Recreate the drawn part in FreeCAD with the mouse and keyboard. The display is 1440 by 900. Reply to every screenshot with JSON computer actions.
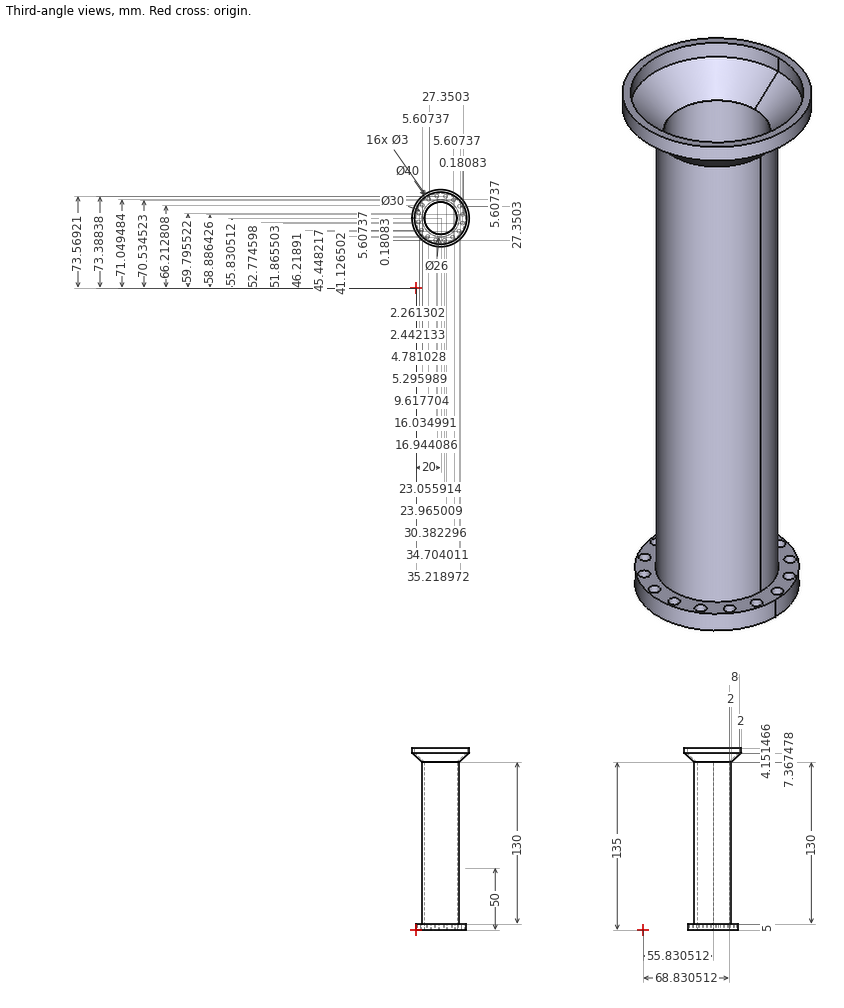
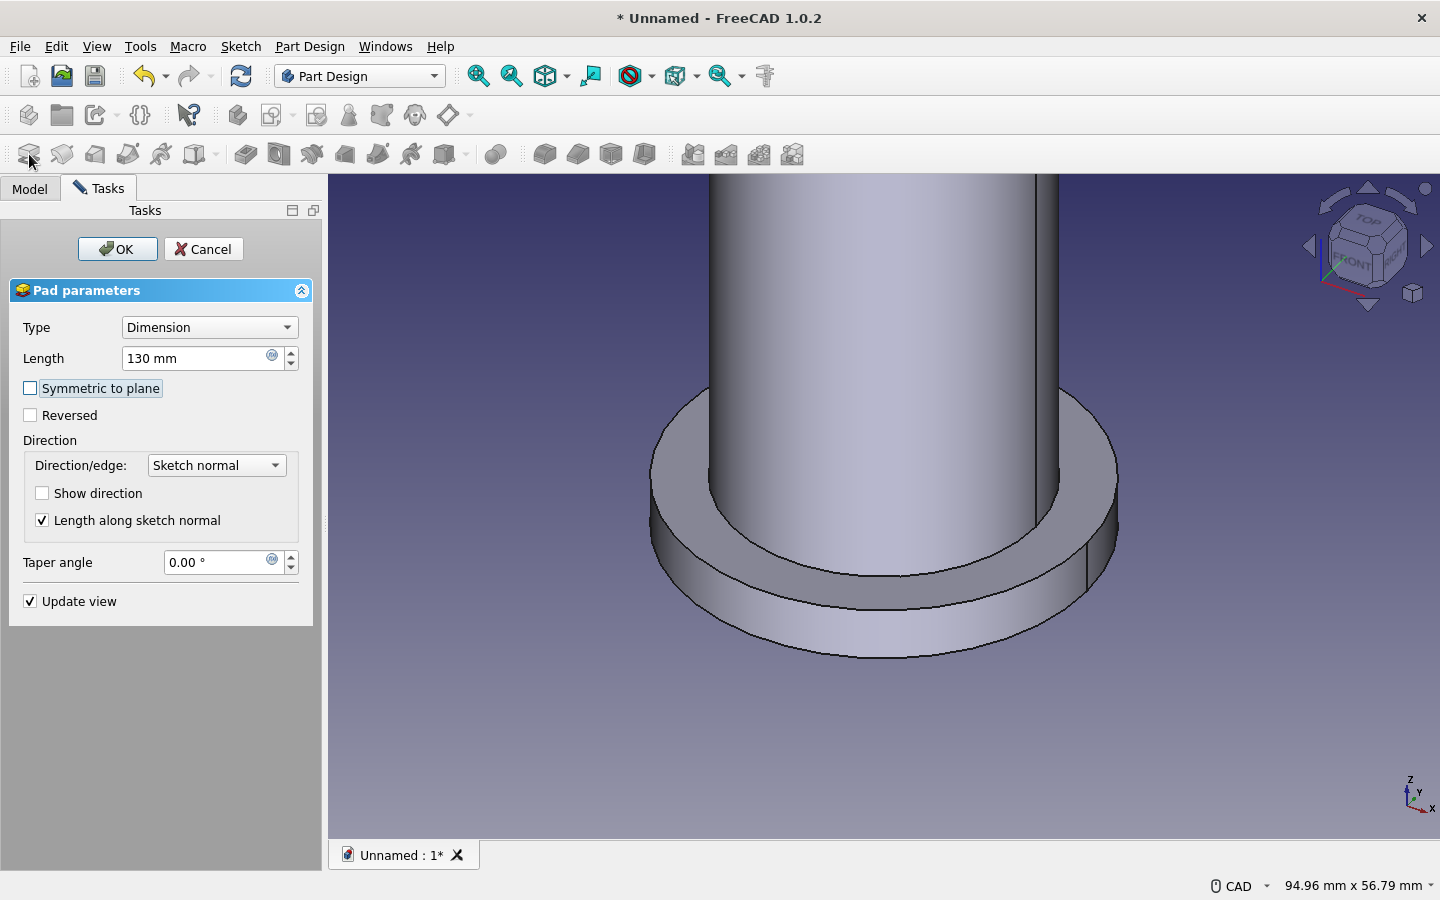
{"action": "left_click", "coordinate": [118, 249]}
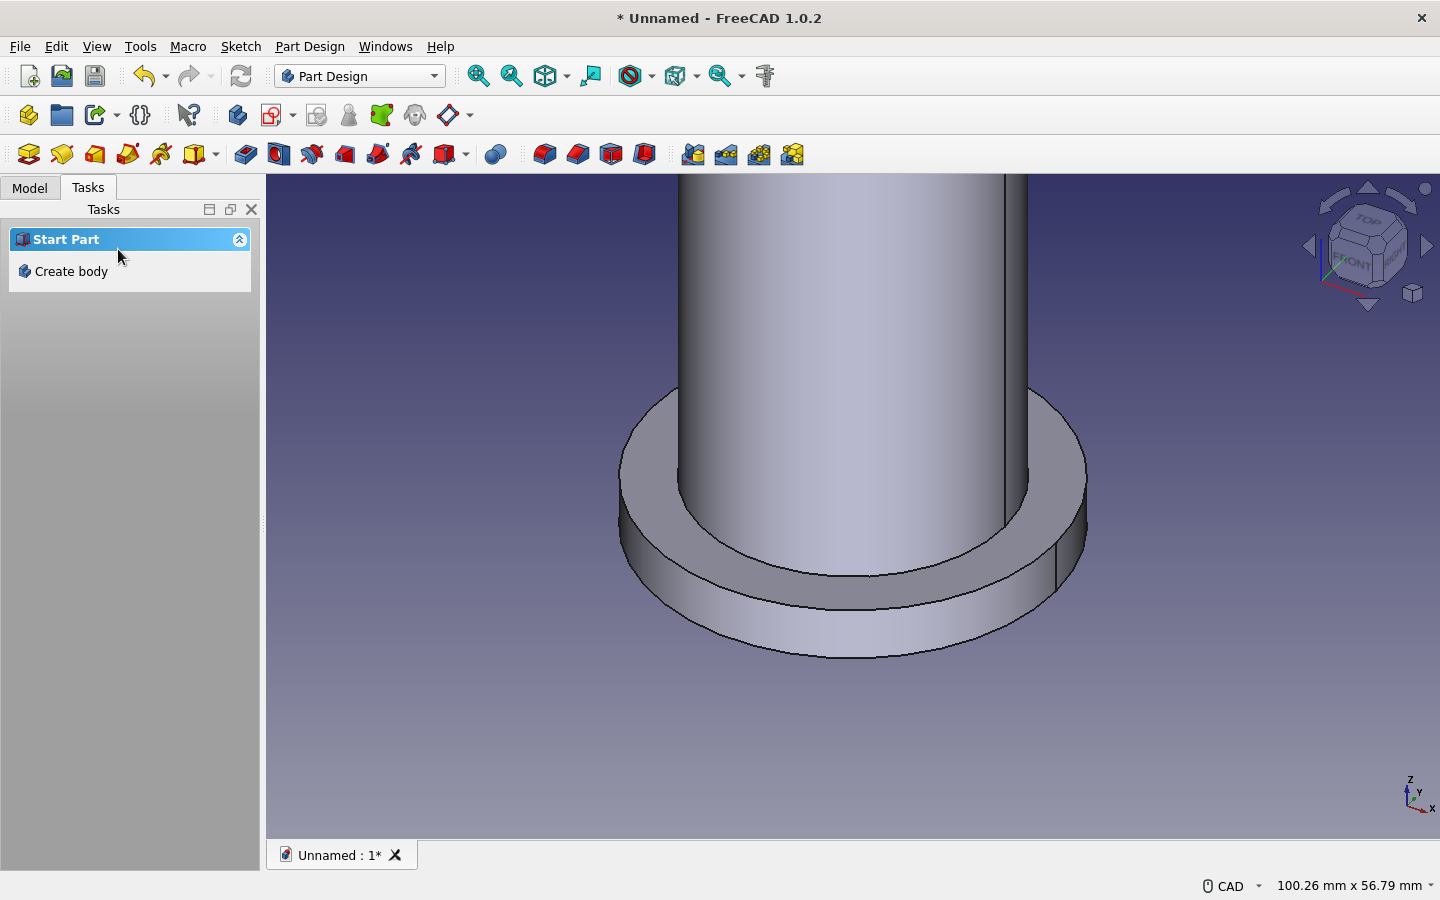
{"action": "left_click", "coordinate": [479, 76]}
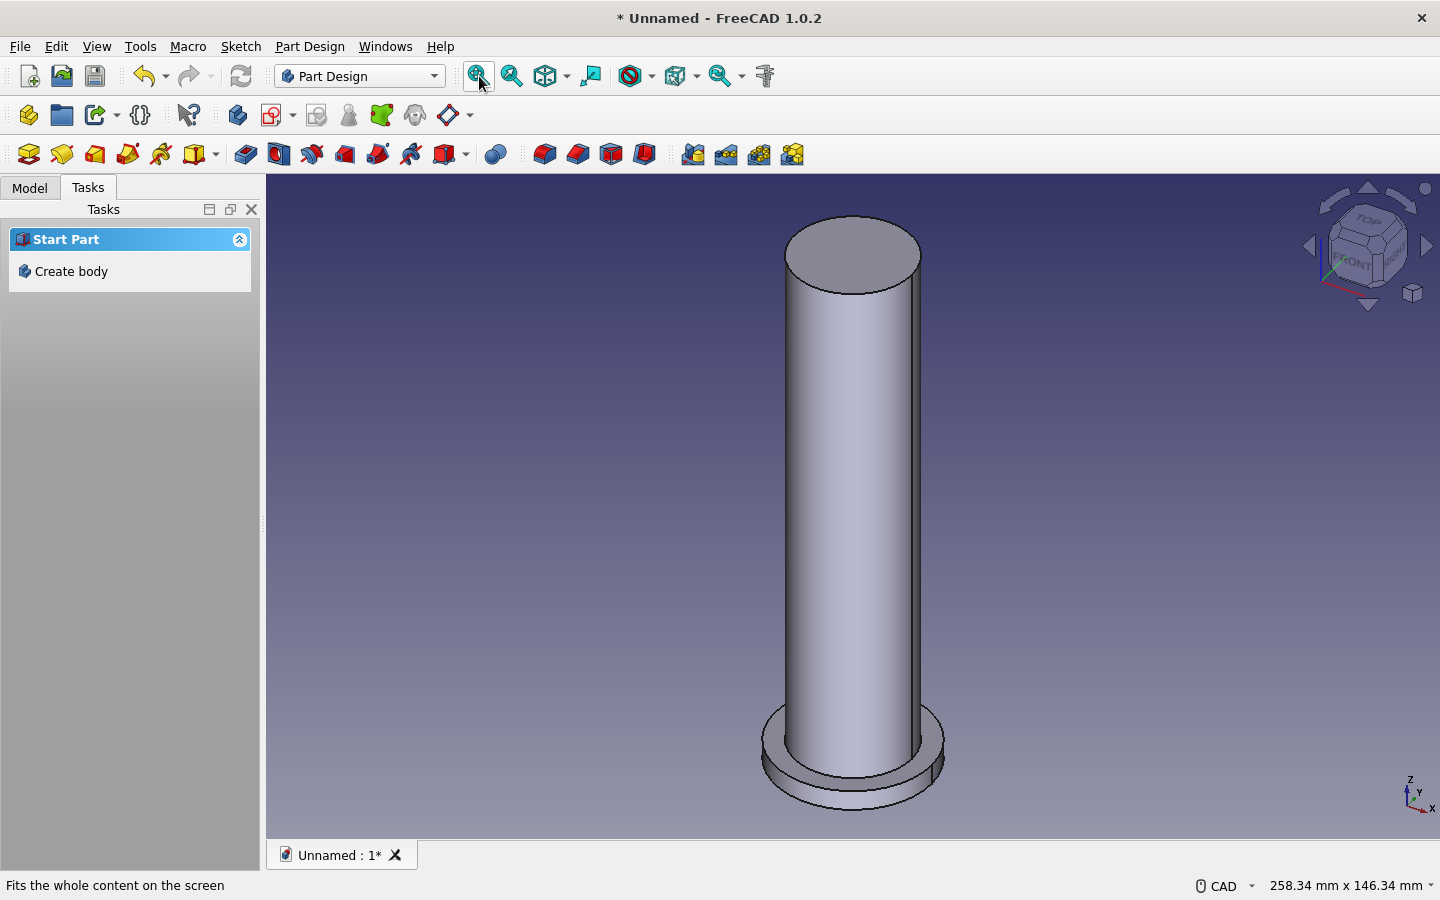
{"action": "left_click", "coordinate": [853, 254]}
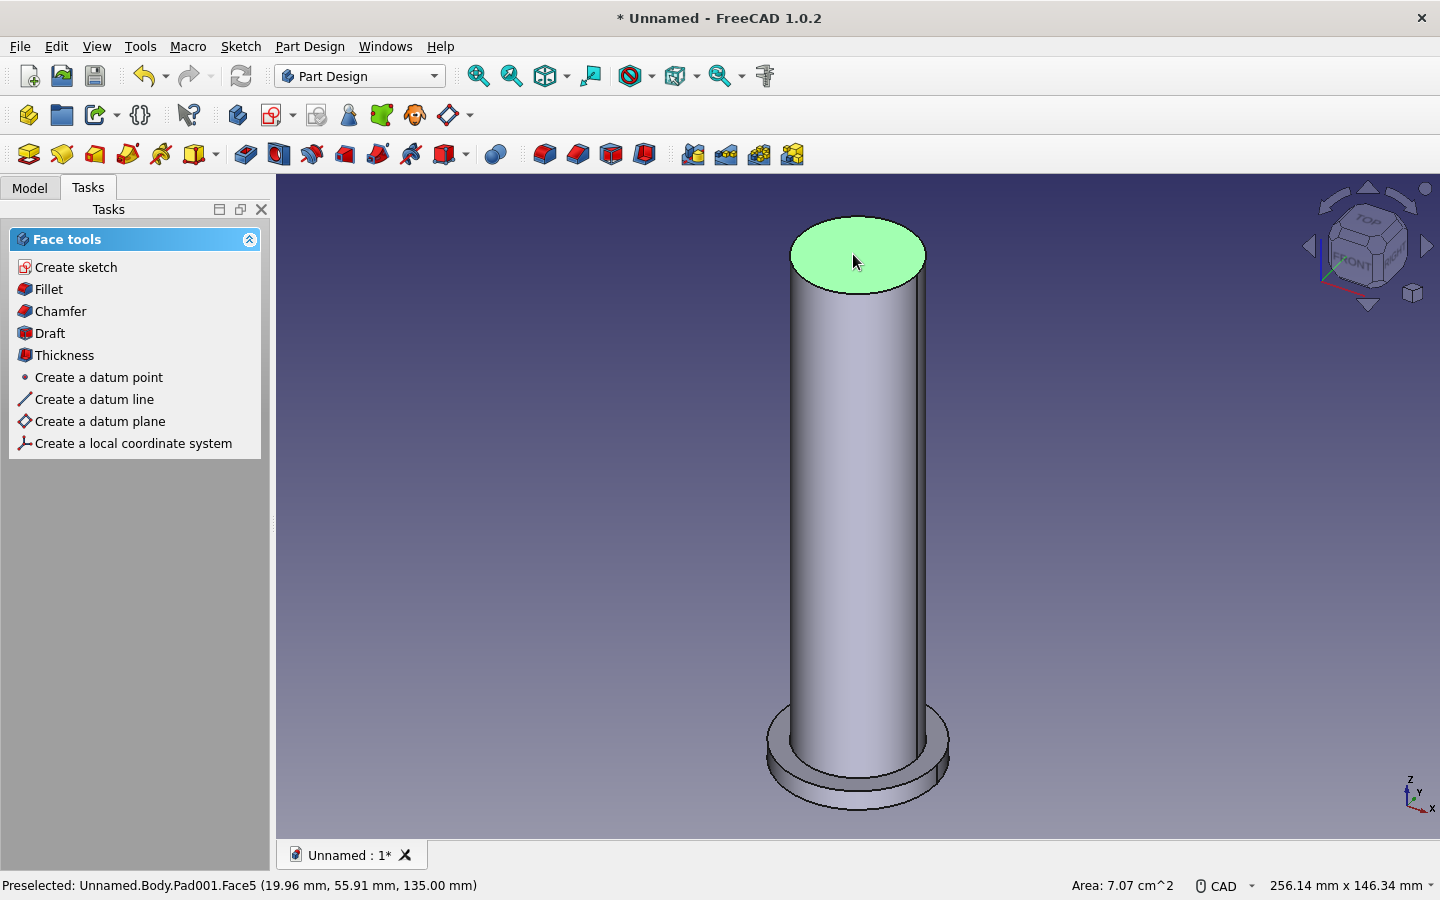
{"action": "left_click", "coordinate": [270, 116]}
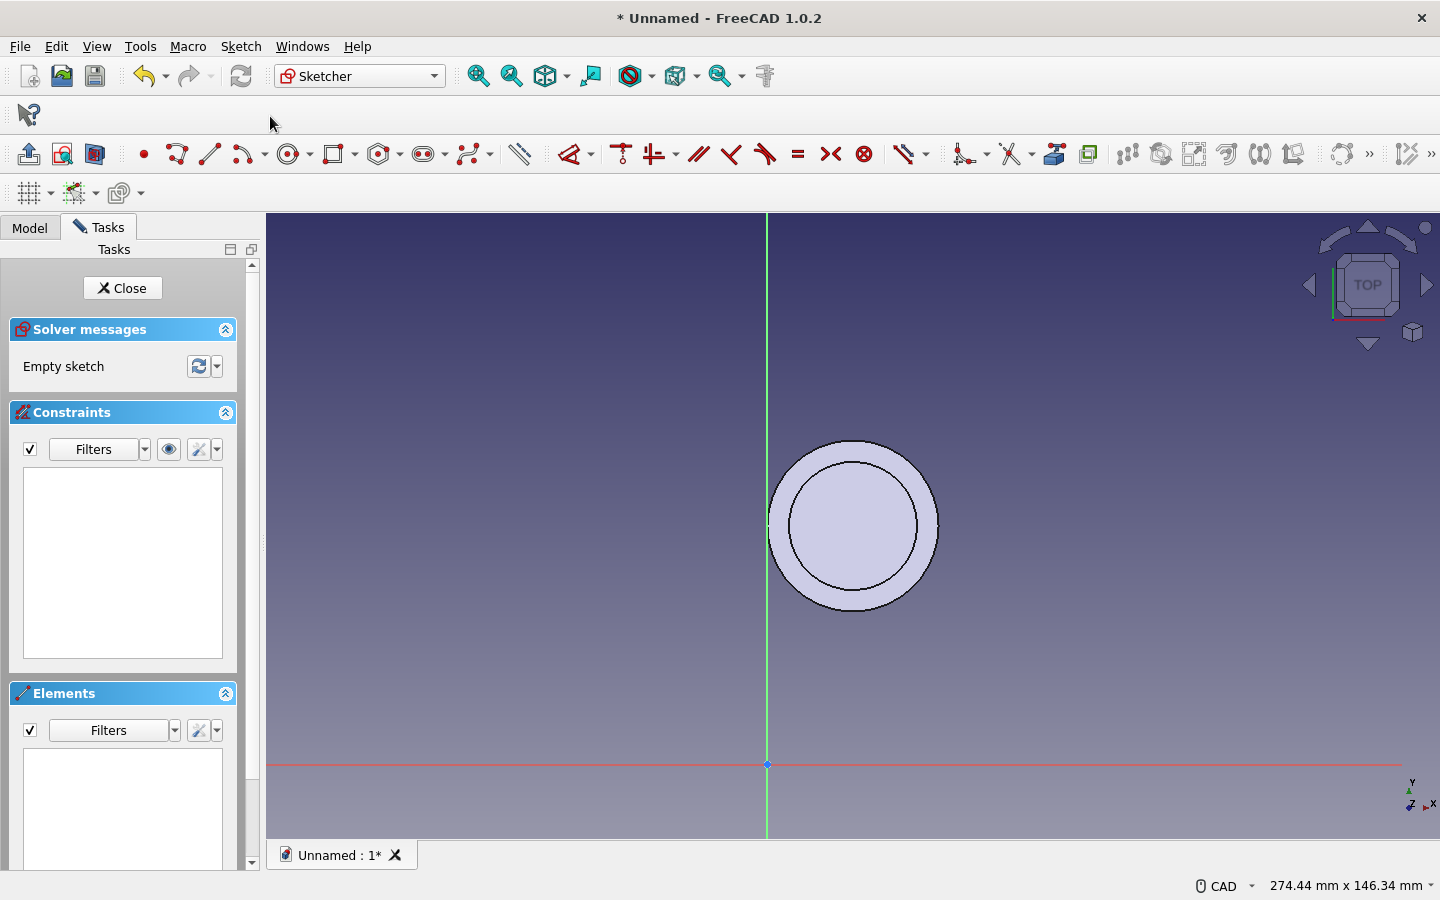
{"action": "scroll", "coordinate": [883, 526], "scroll_direction": "up", "scroll_amount": 6}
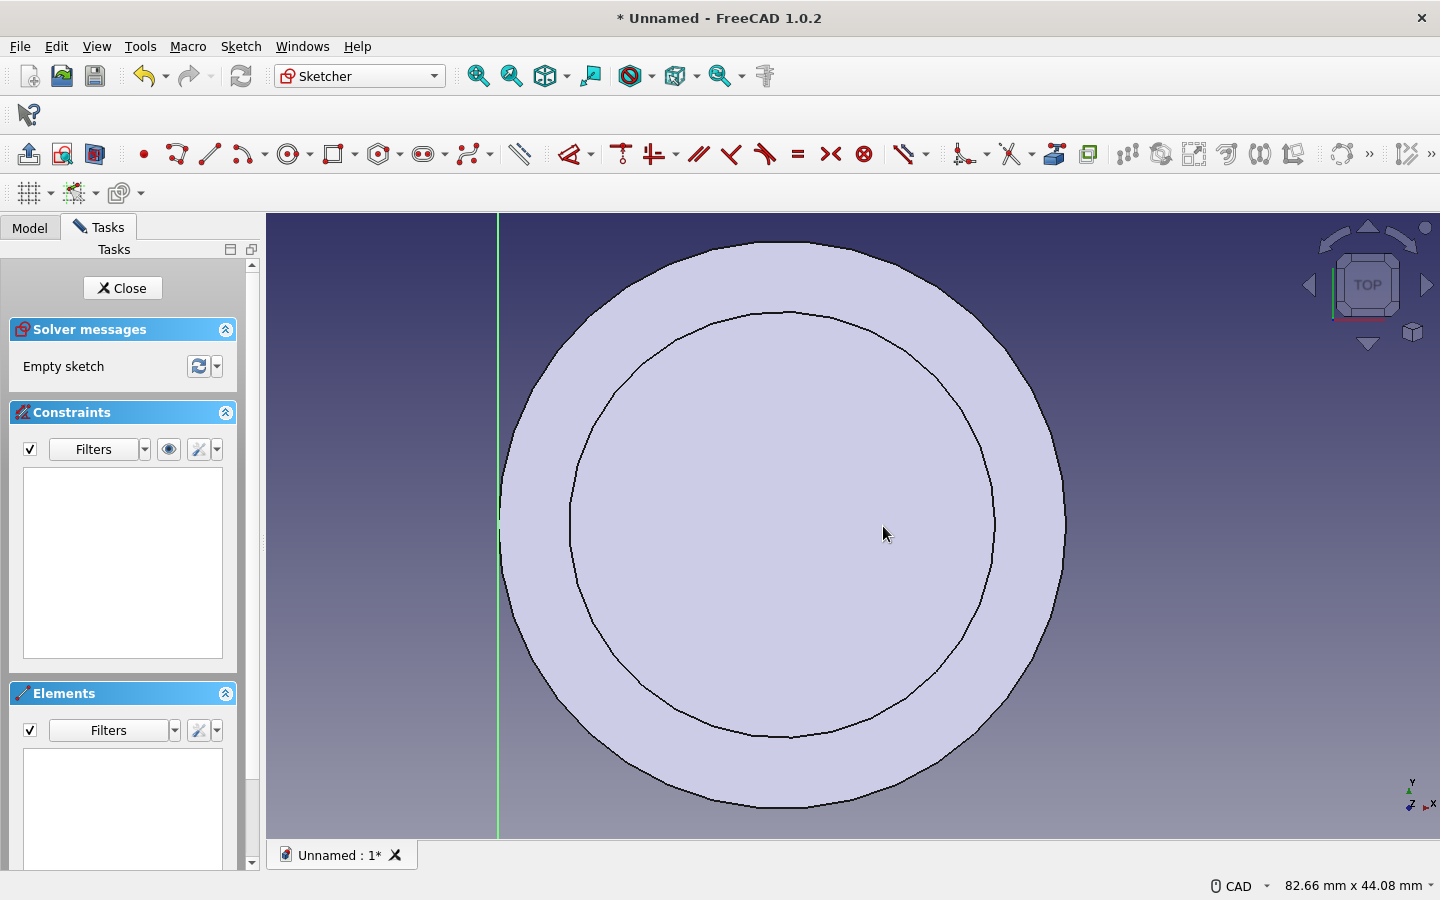
{"action": "key", "text": "g c"}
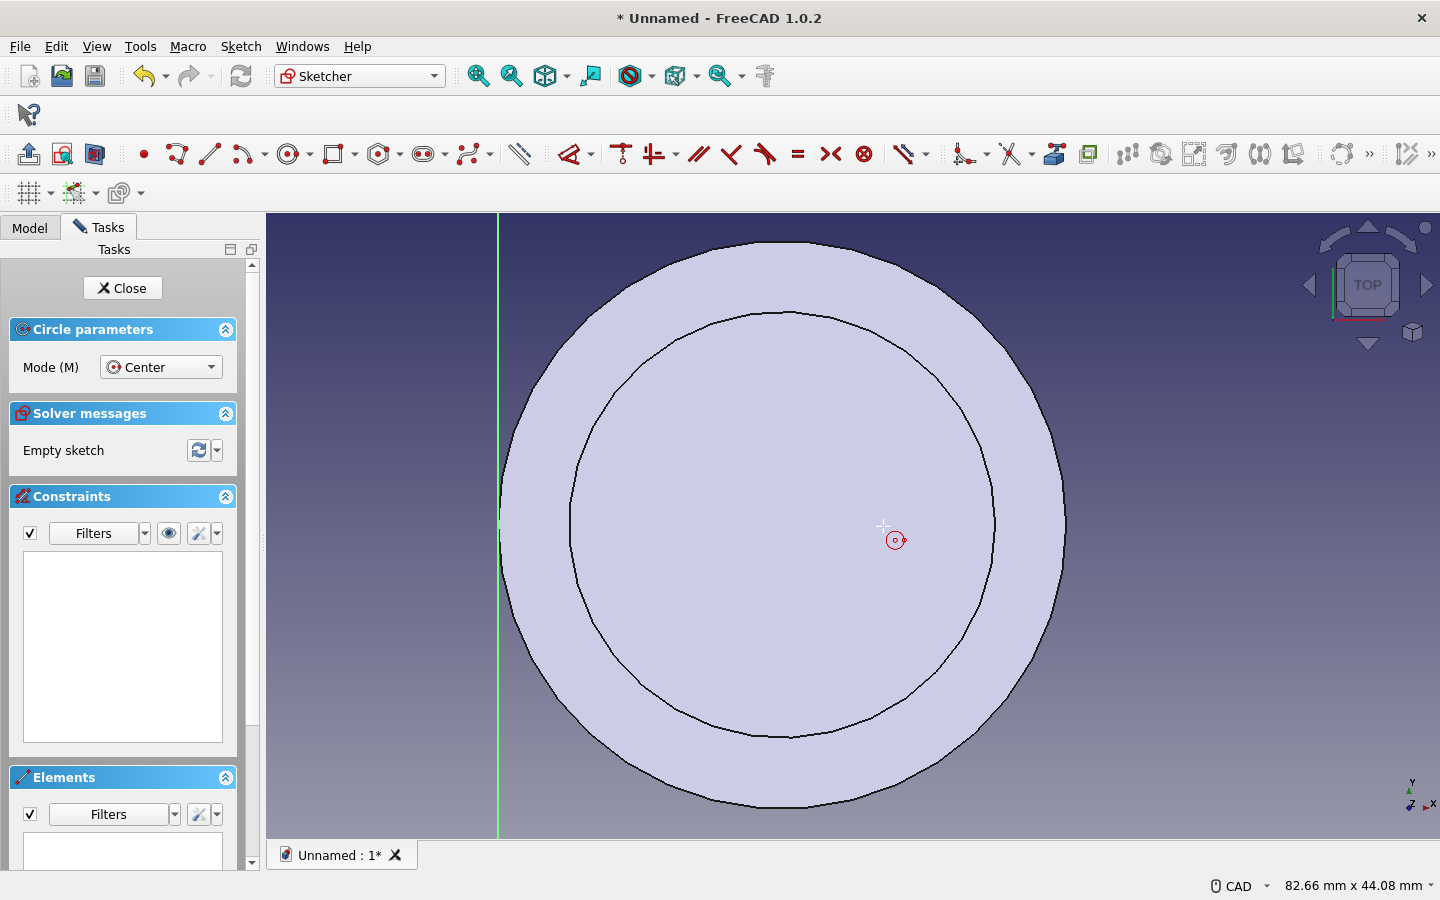
{"action": "left_click", "coordinate": [782, 525]}
{"action": "mouse_move", "coordinate": [913, 394]}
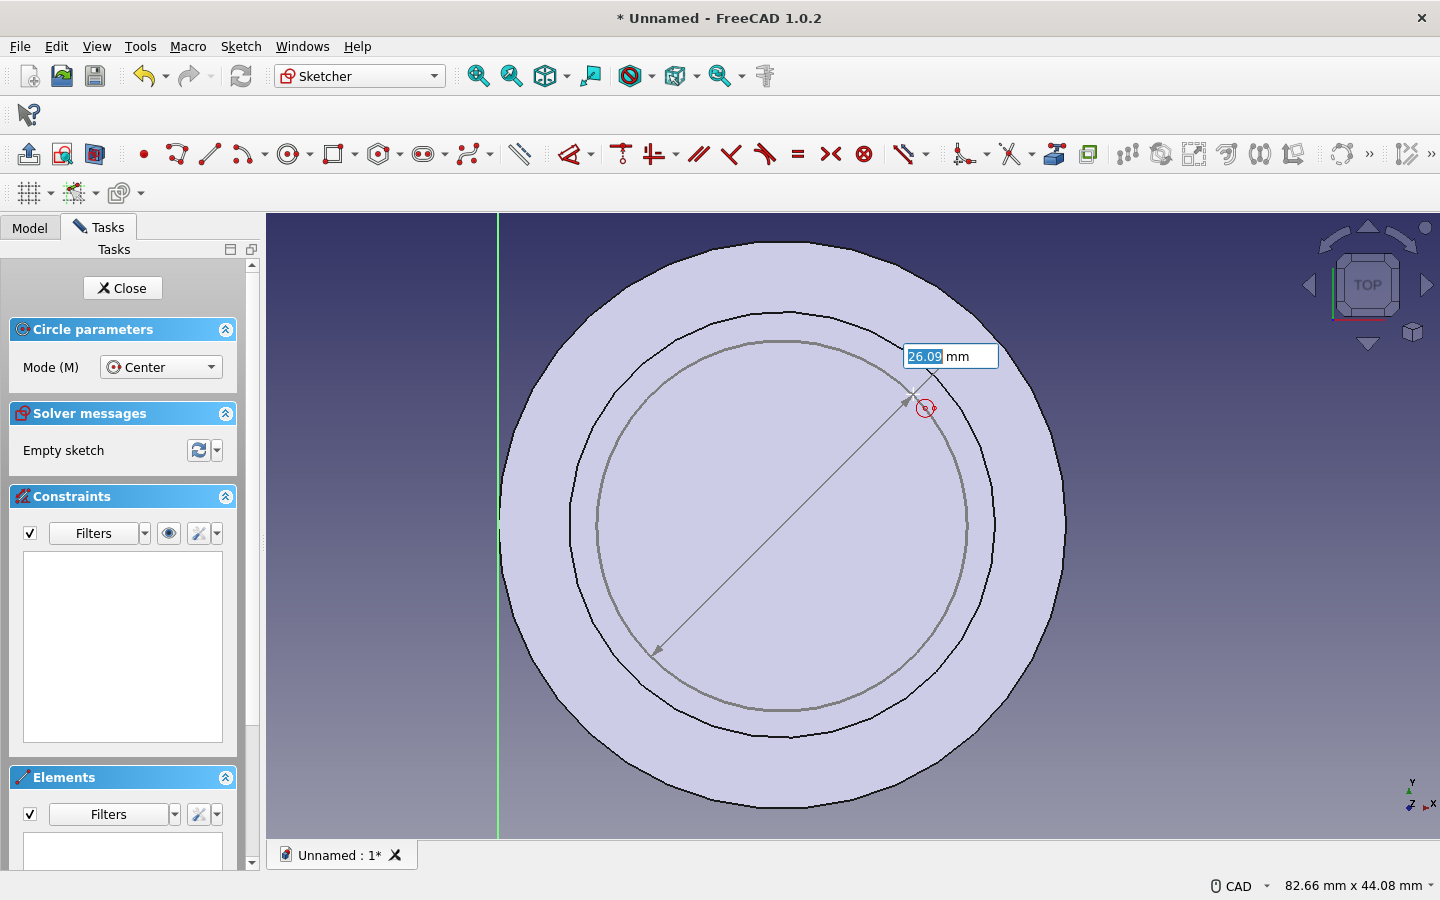
{"action": "type", "text": "26"}
{"action": "key", "text": "Return"}
{"action": "key", "text": "Escape"}